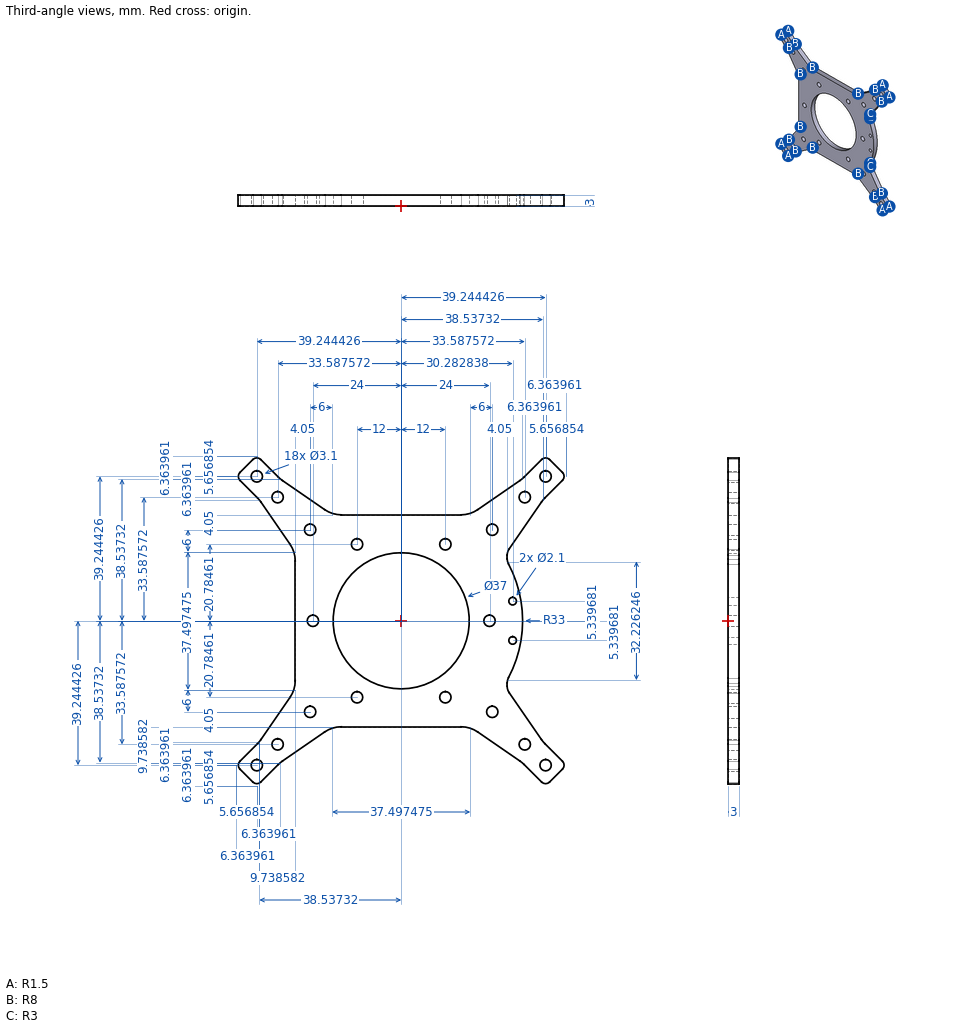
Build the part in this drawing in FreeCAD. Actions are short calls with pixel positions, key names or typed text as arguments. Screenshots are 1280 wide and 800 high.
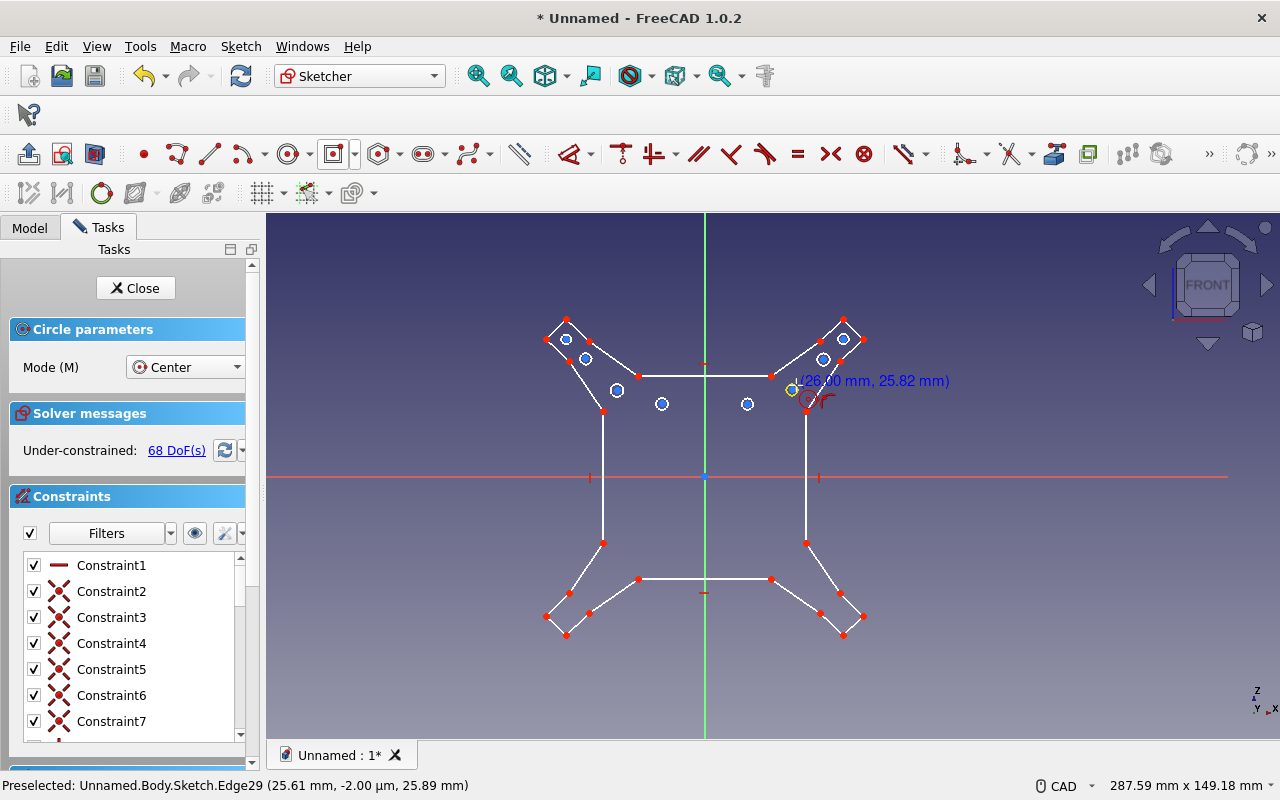
scroll(620, 477, up, 8)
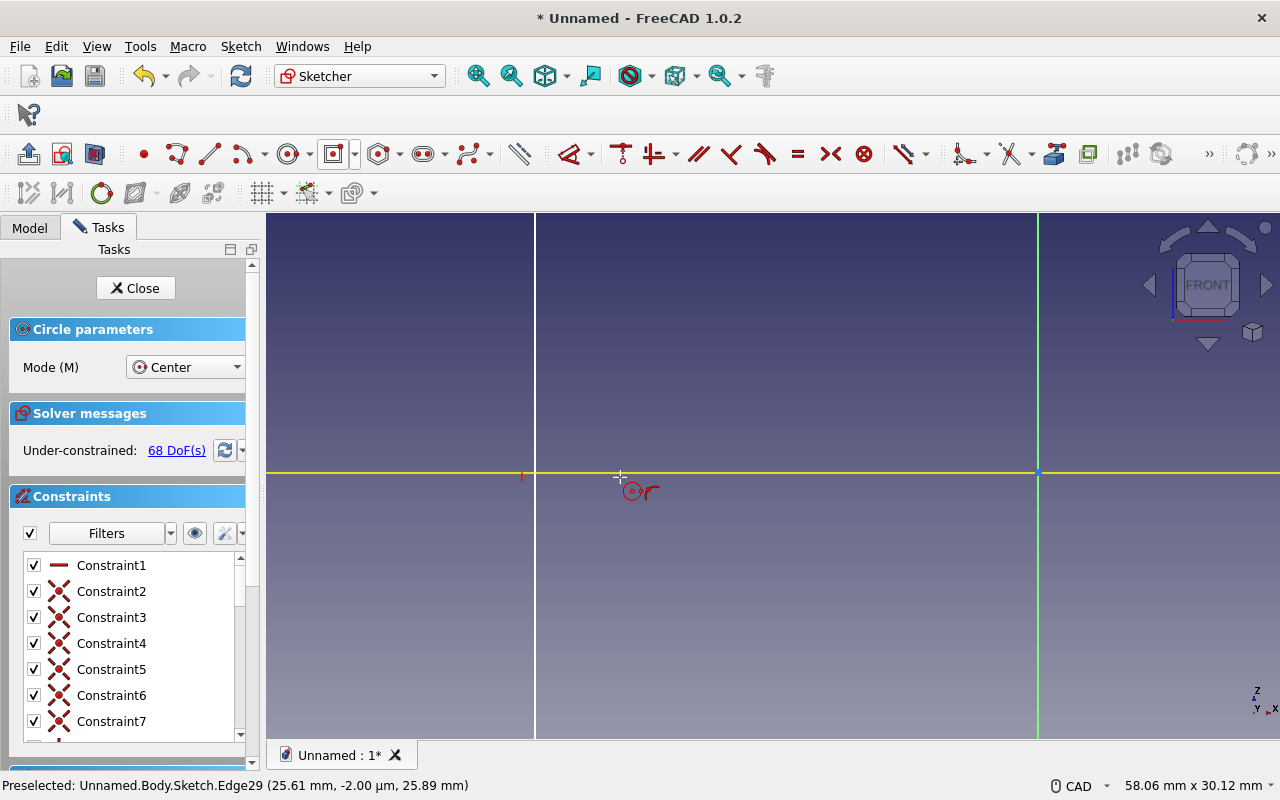
scroll(620, 477, down, 8)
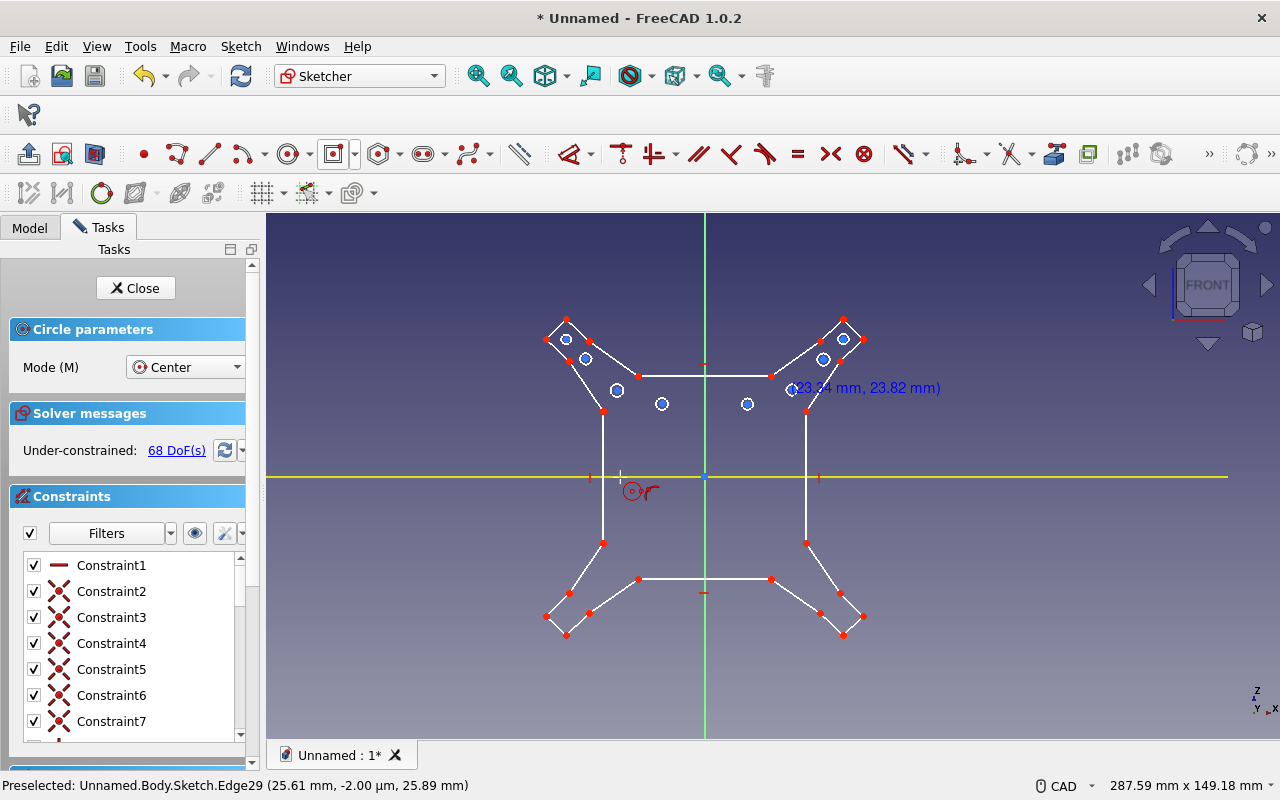
click(620, 477)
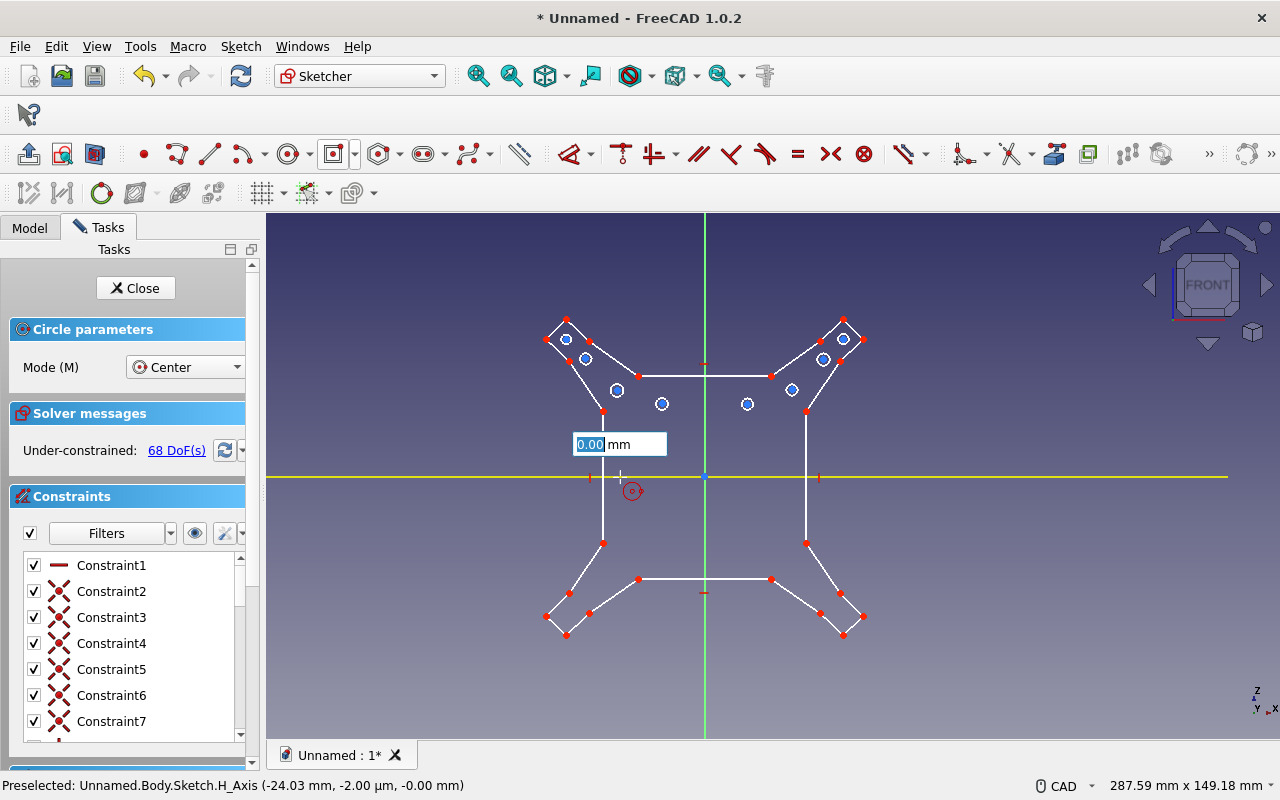
scroll(622, 471, up, 6)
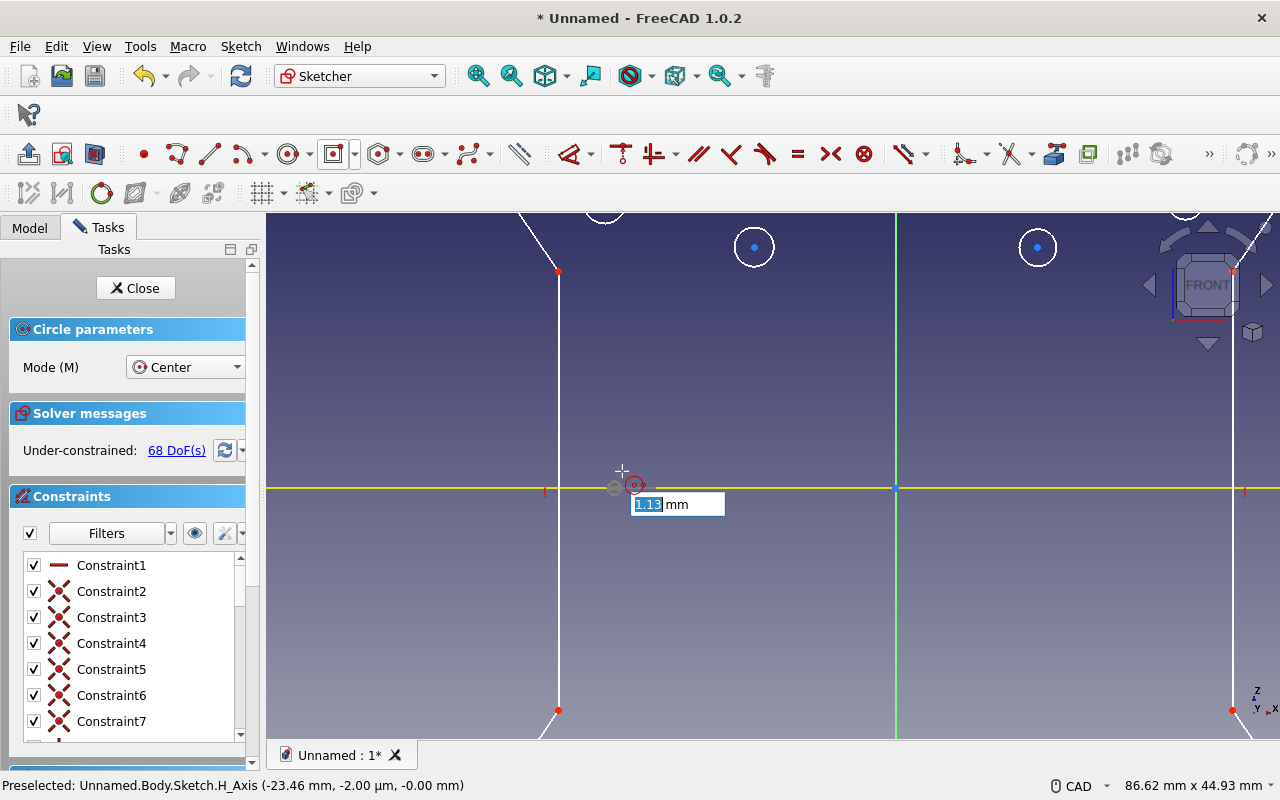
click(621, 471)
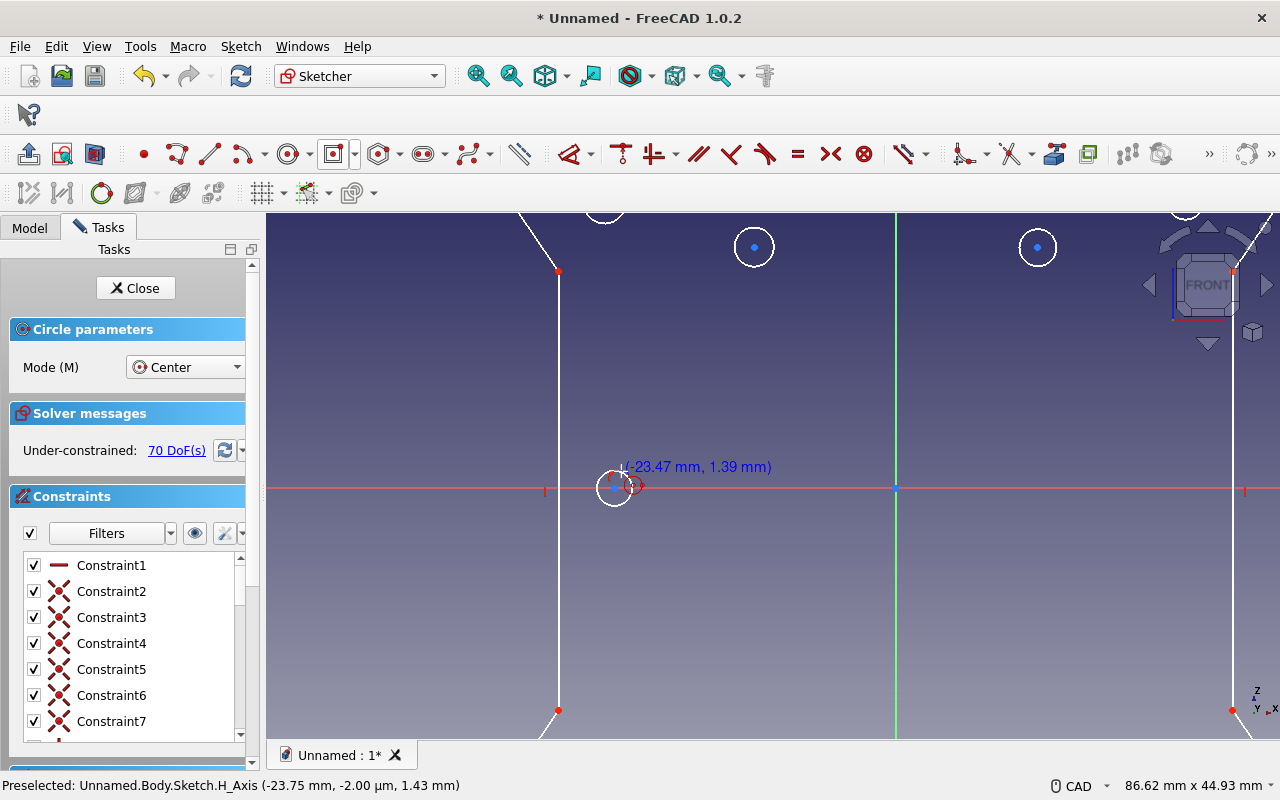
scroll(622, 471, down, 6)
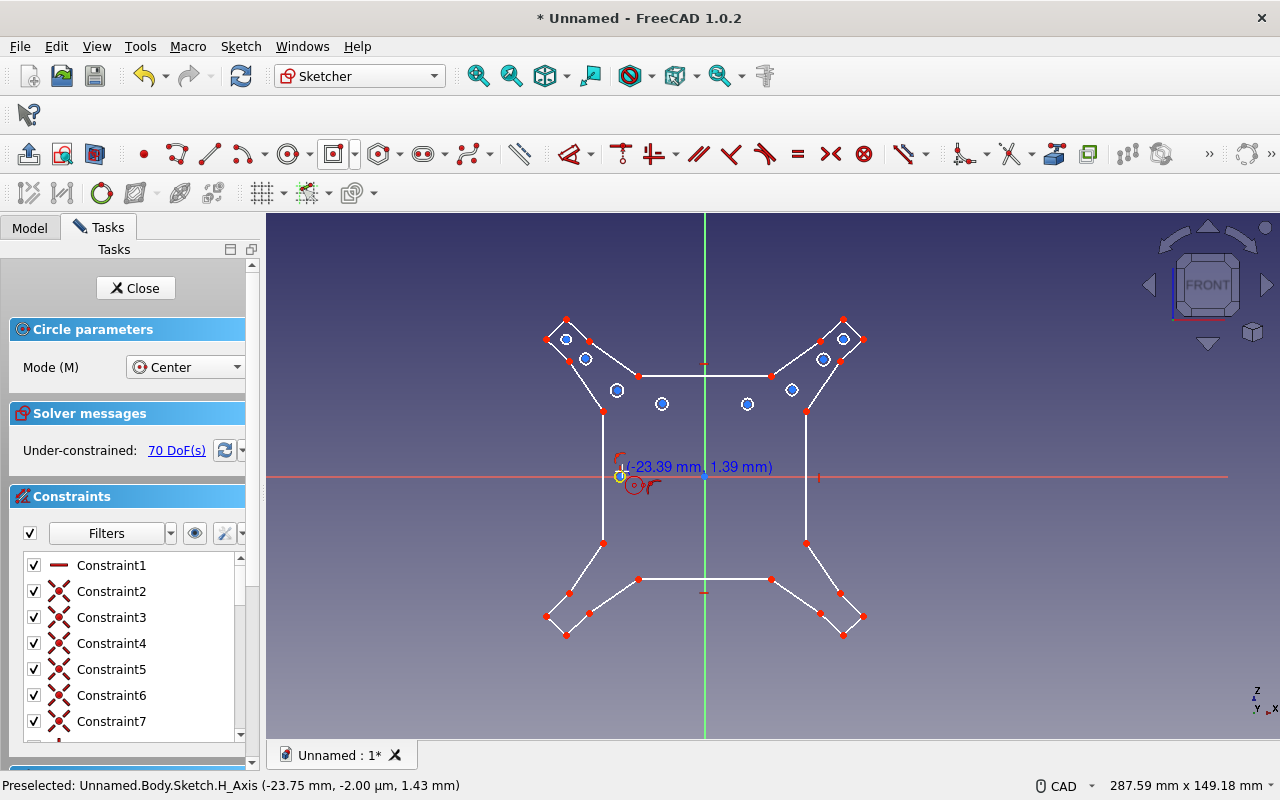
scroll(617, 564, up, 8)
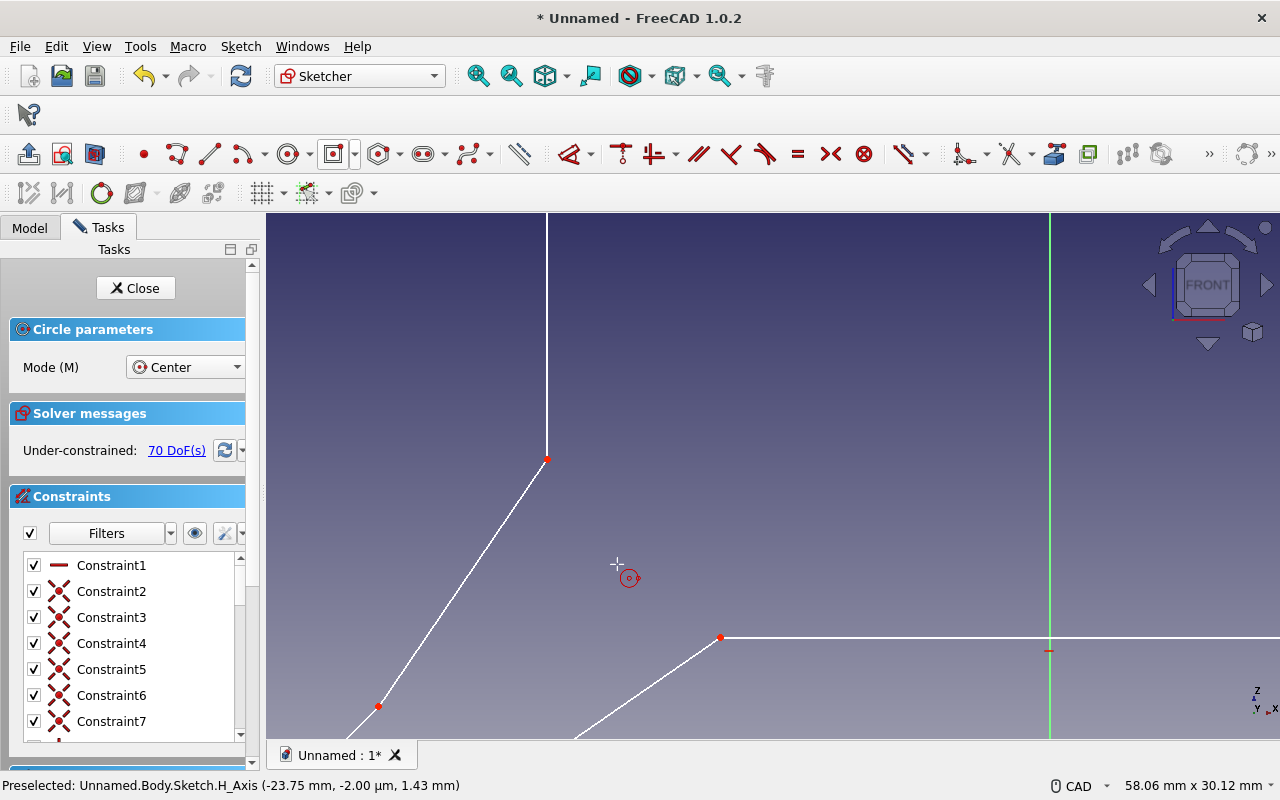
scroll(617, 564, down, 8)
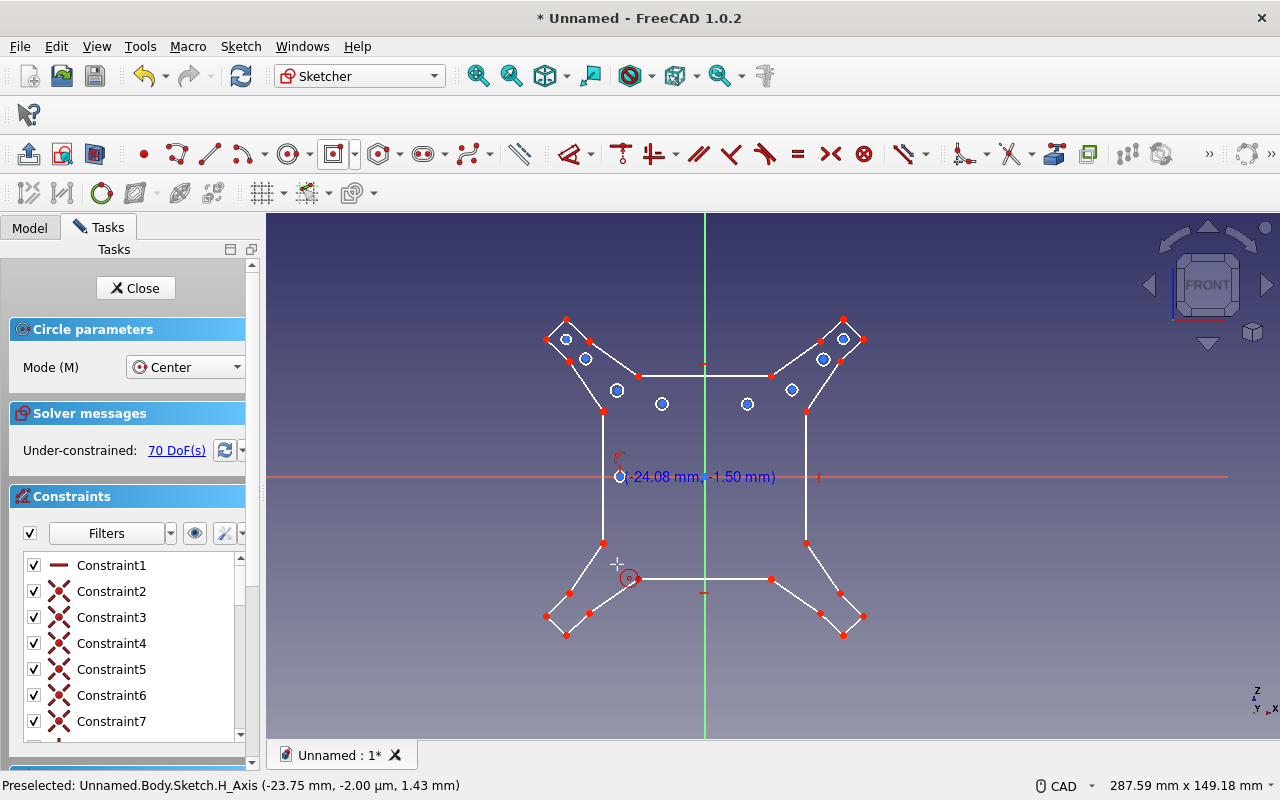
click(617, 564)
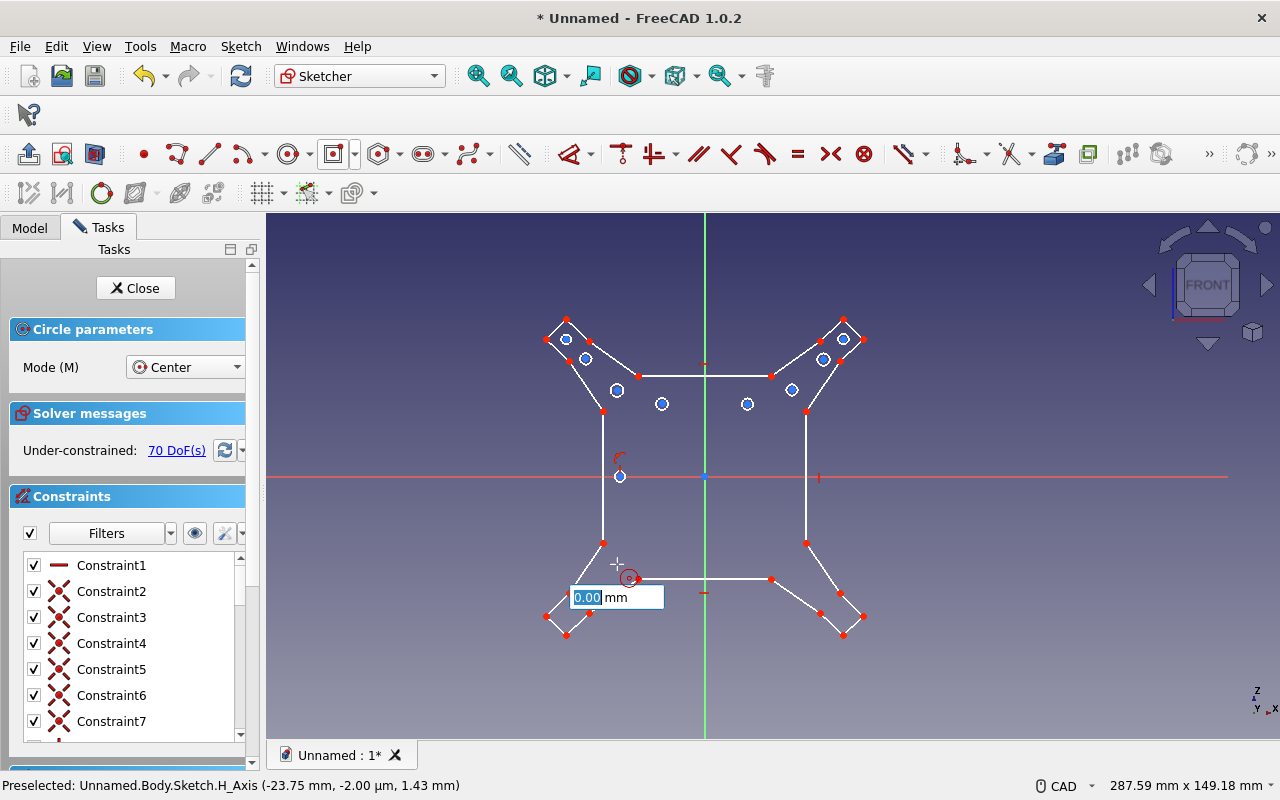
scroll(621, 560, up, 6)